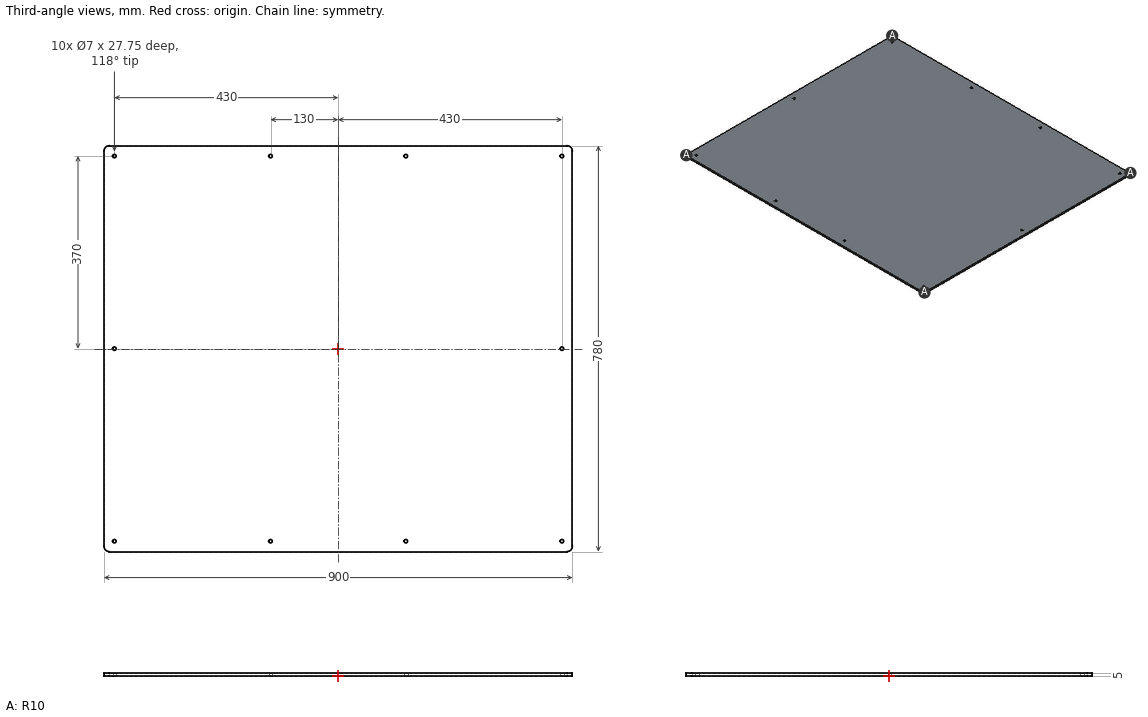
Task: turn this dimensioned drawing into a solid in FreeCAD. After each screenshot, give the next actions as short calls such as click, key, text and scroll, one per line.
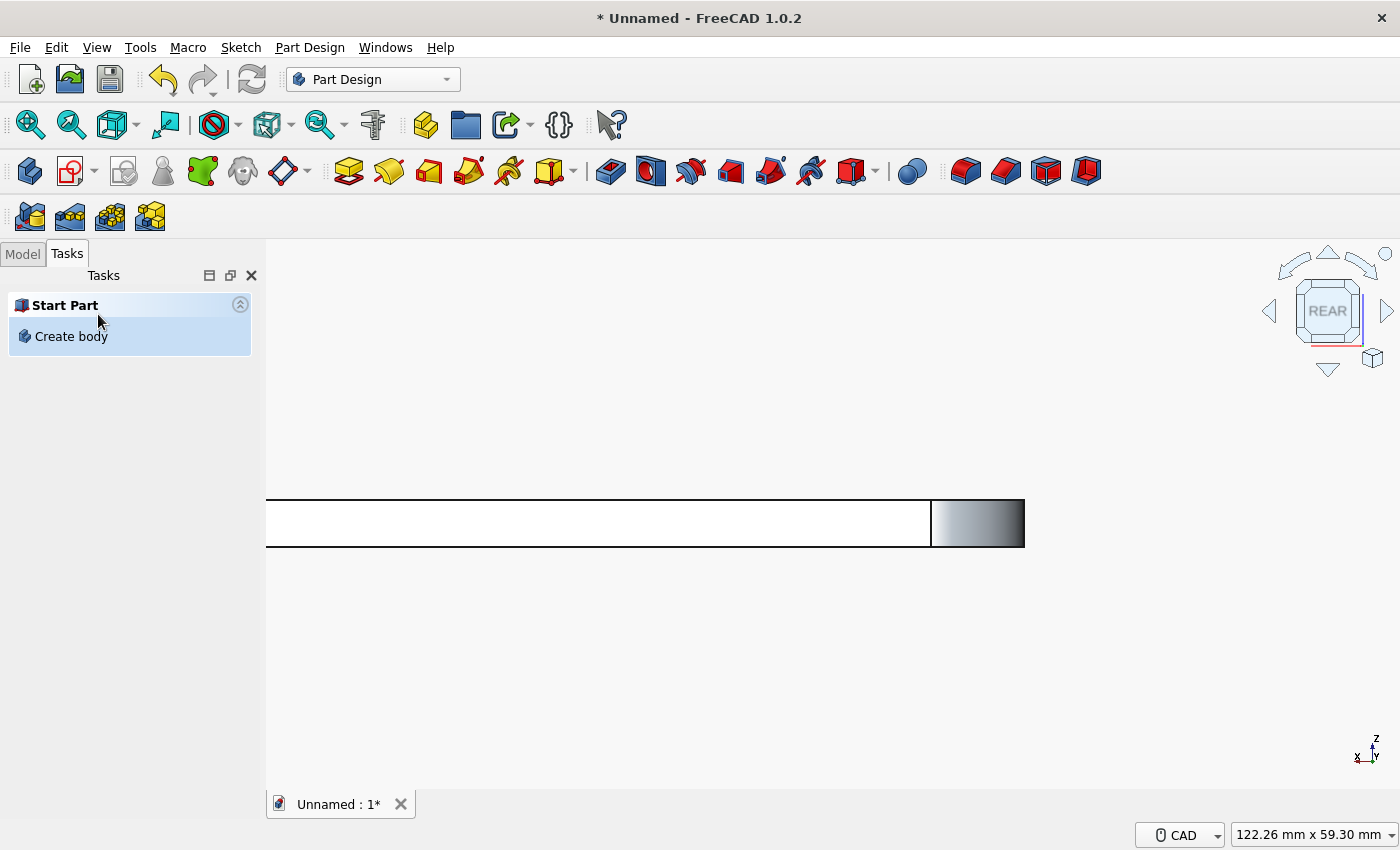
key(0)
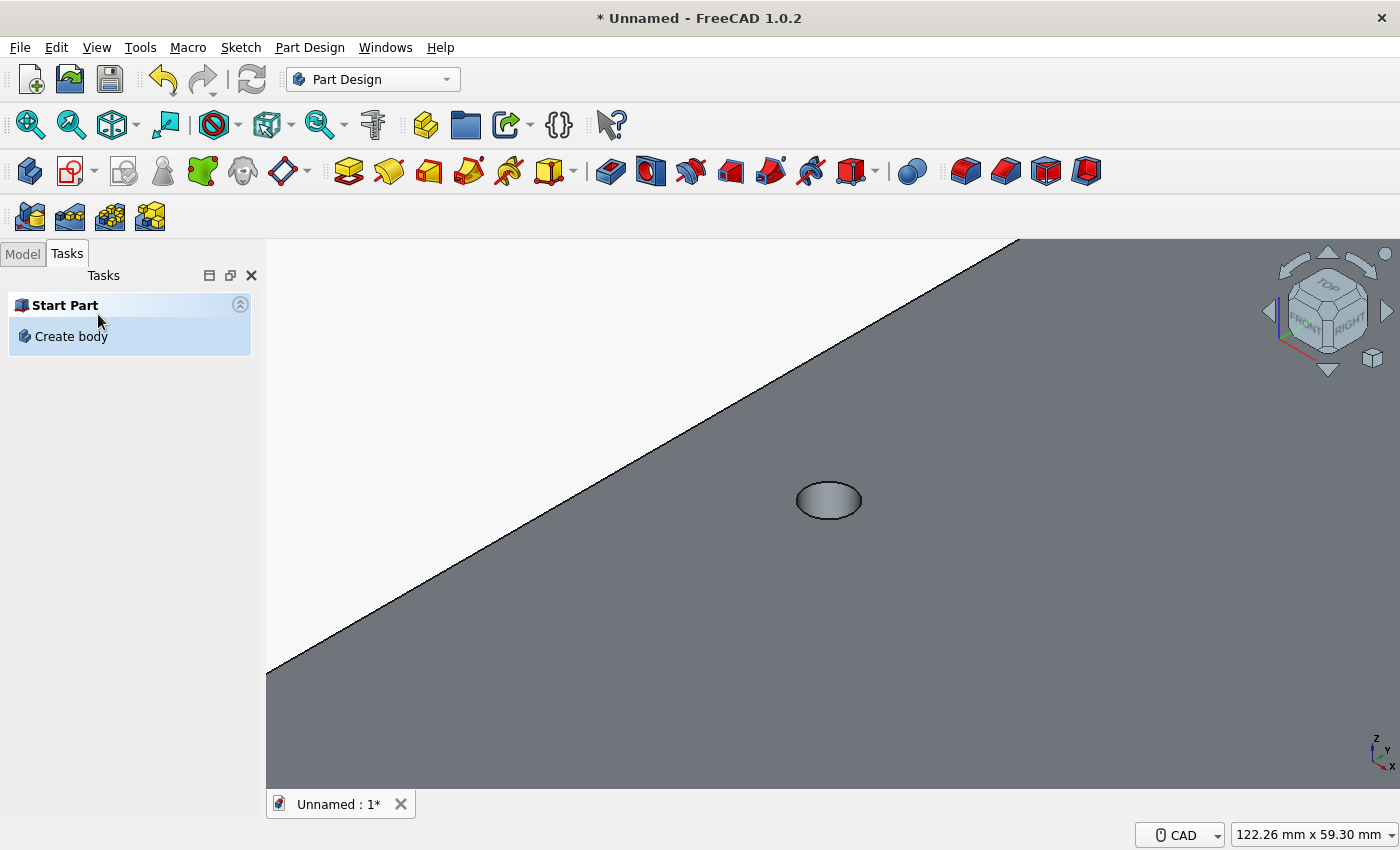
key(v)
key(f)